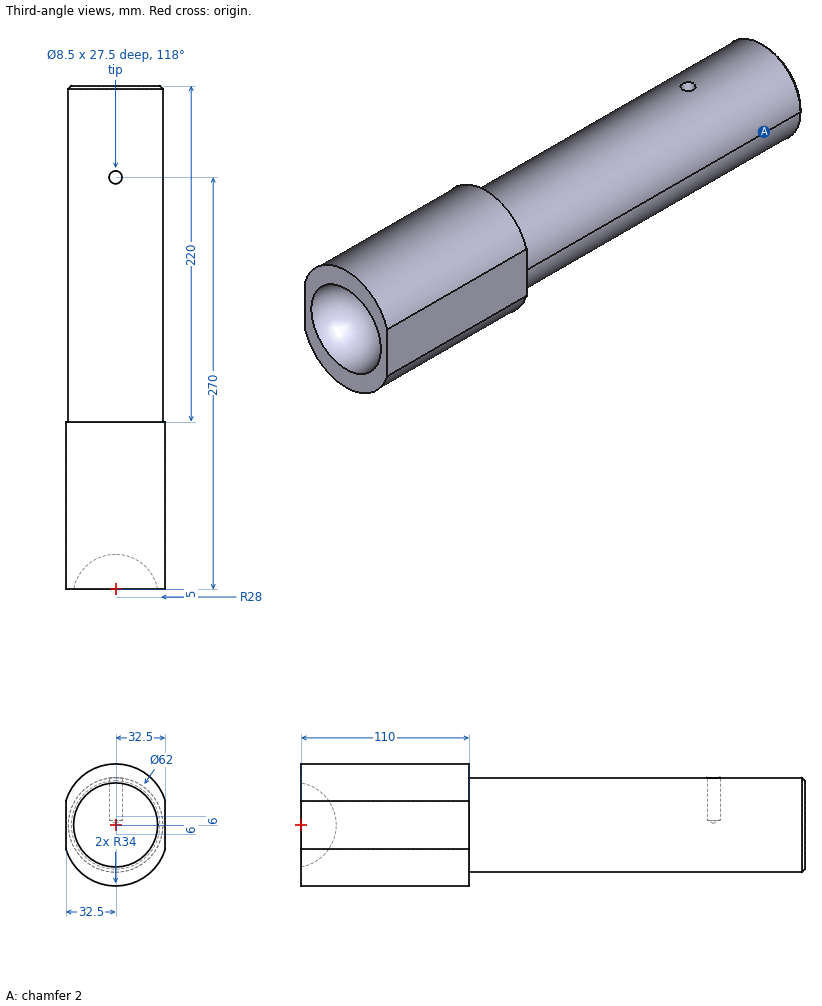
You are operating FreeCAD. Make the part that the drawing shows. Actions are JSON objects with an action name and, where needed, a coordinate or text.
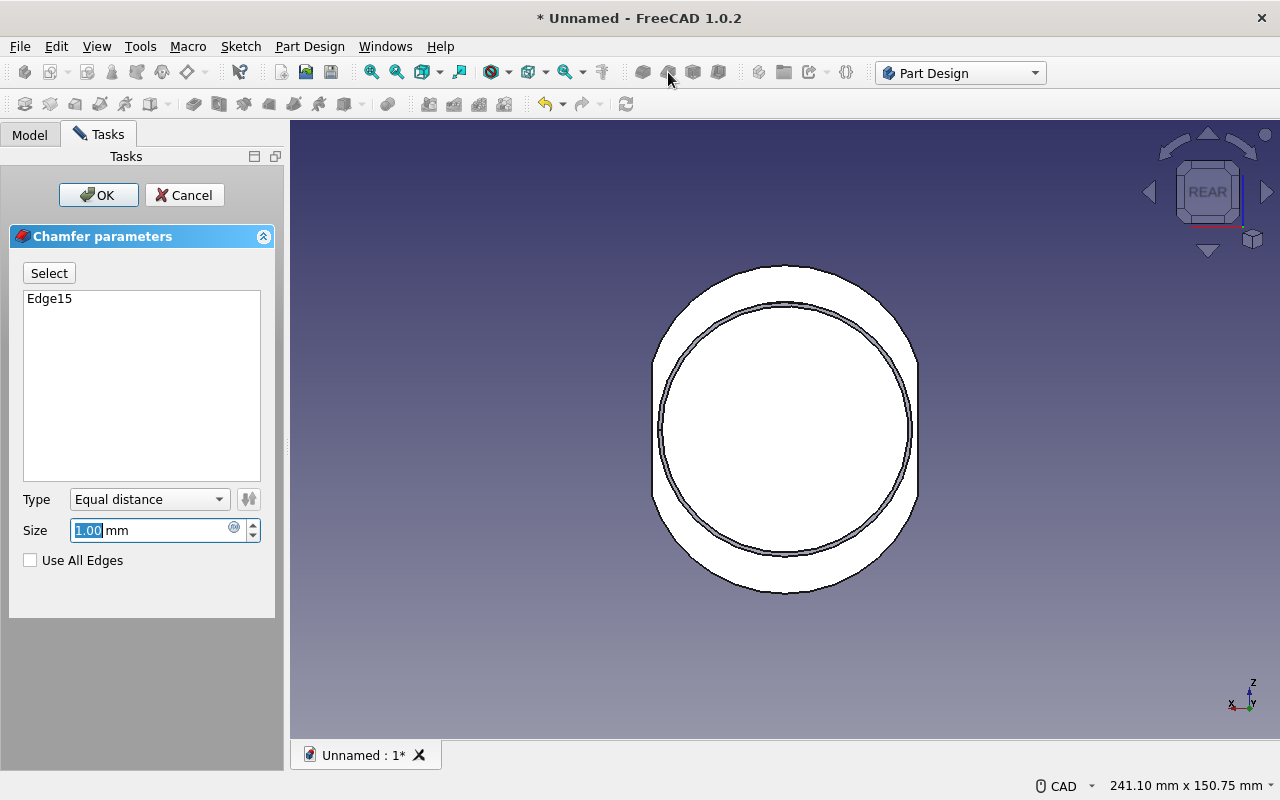
{"action": "type", "text": "2"}
{"action": "key", "text": "Tab"}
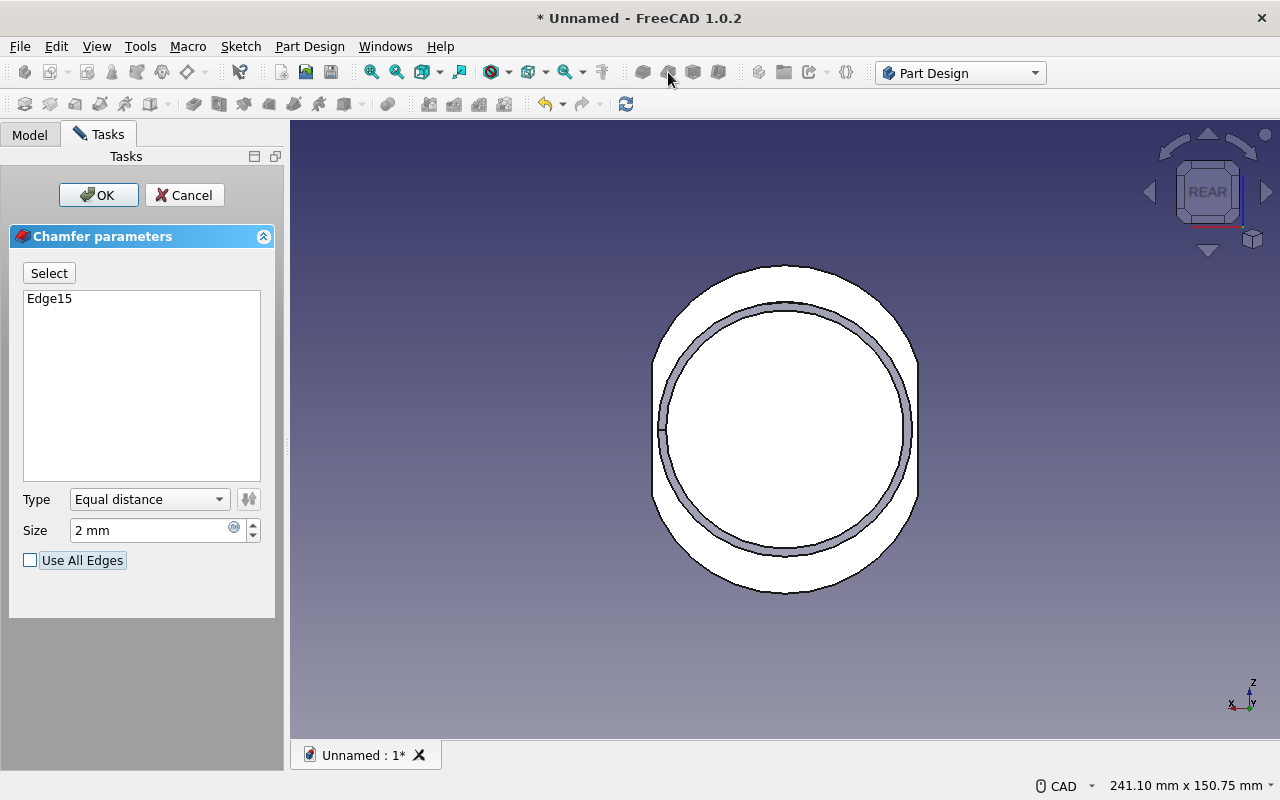
{"action": "left_click", "coordinate": [99, 195]}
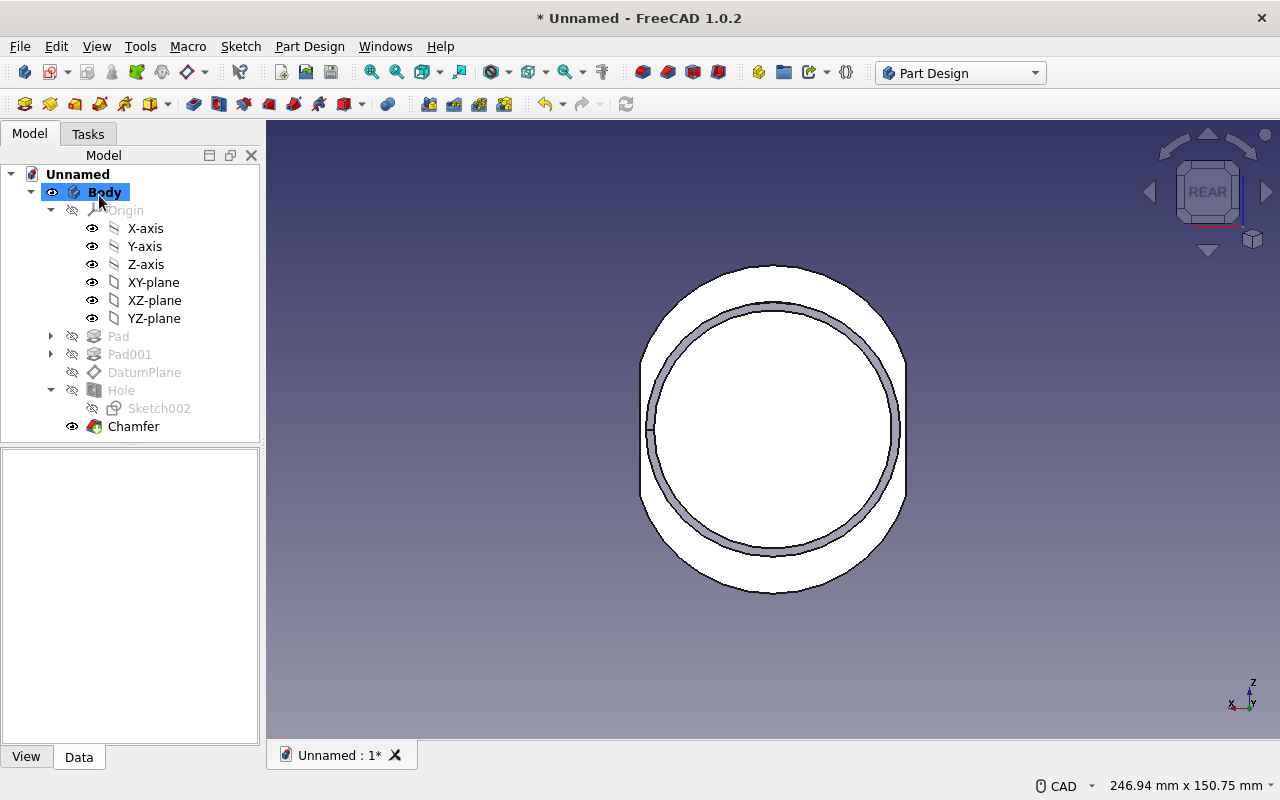
{"action": "left_click", "coordinate": [50, 72]}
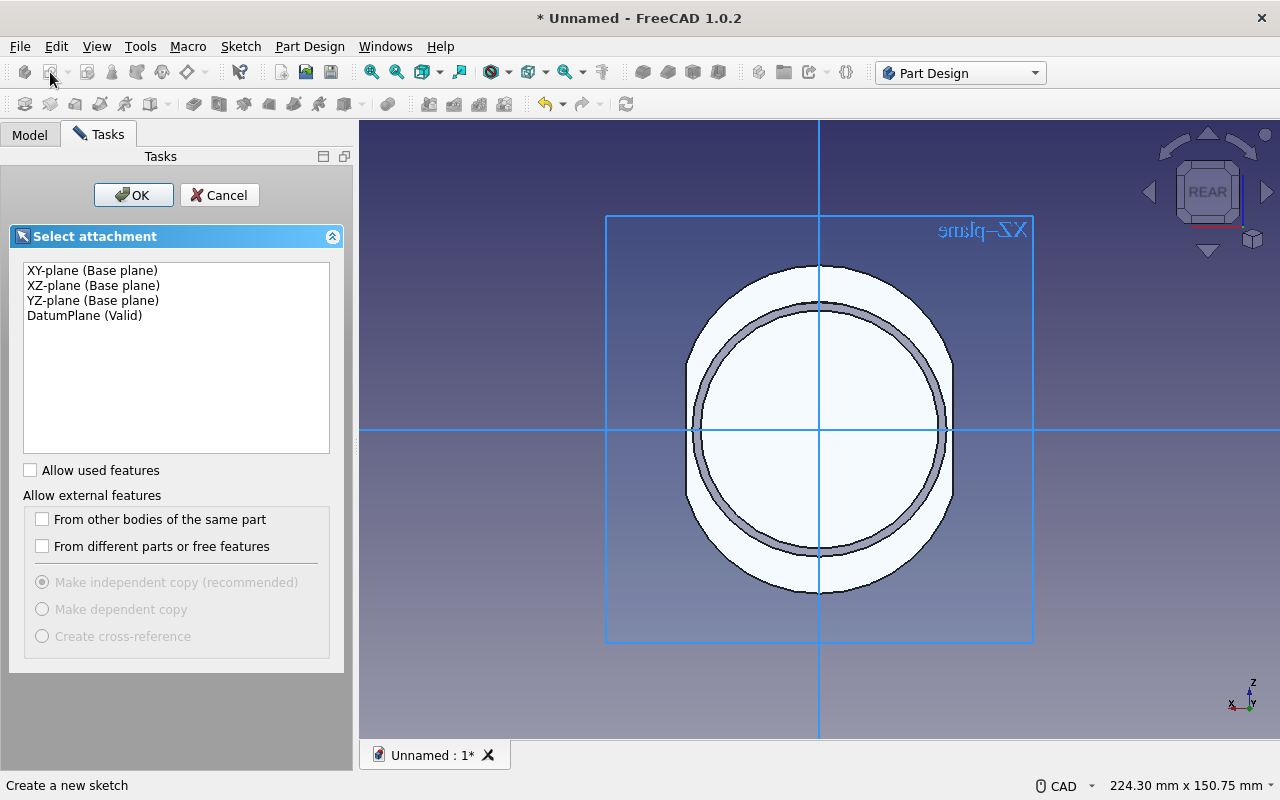
{"action": "left_click", "coordinate": [84, 270]}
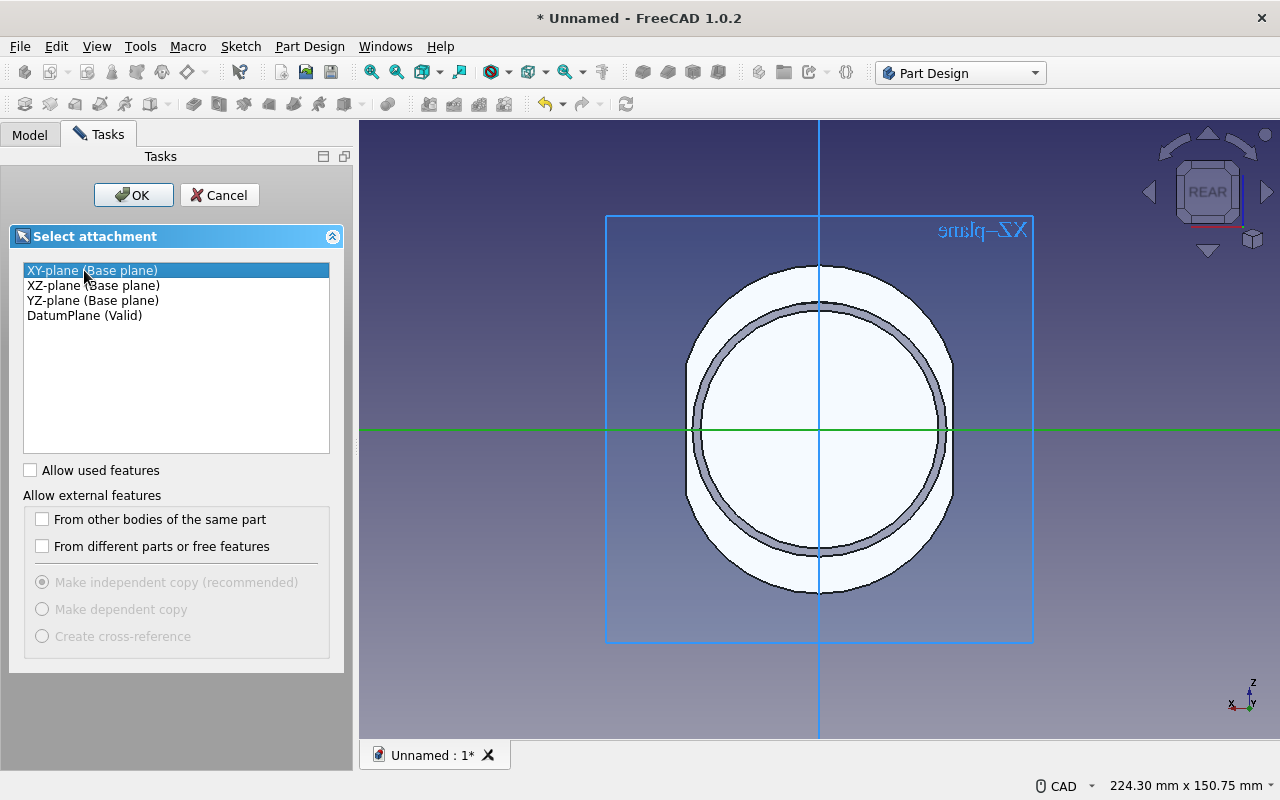
{"action": "left_click", "coordinate": [134, 195]}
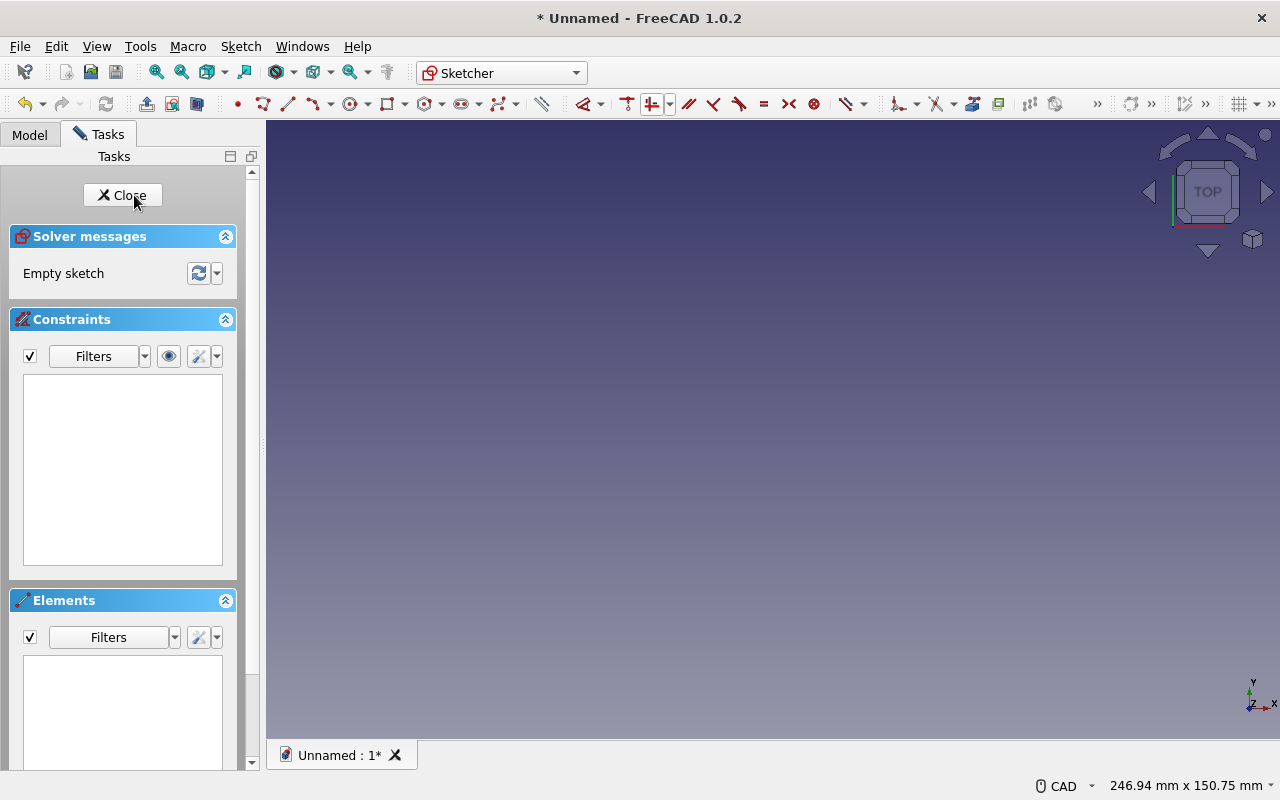
{"action": "left_click", "coordinate": [197, 104]}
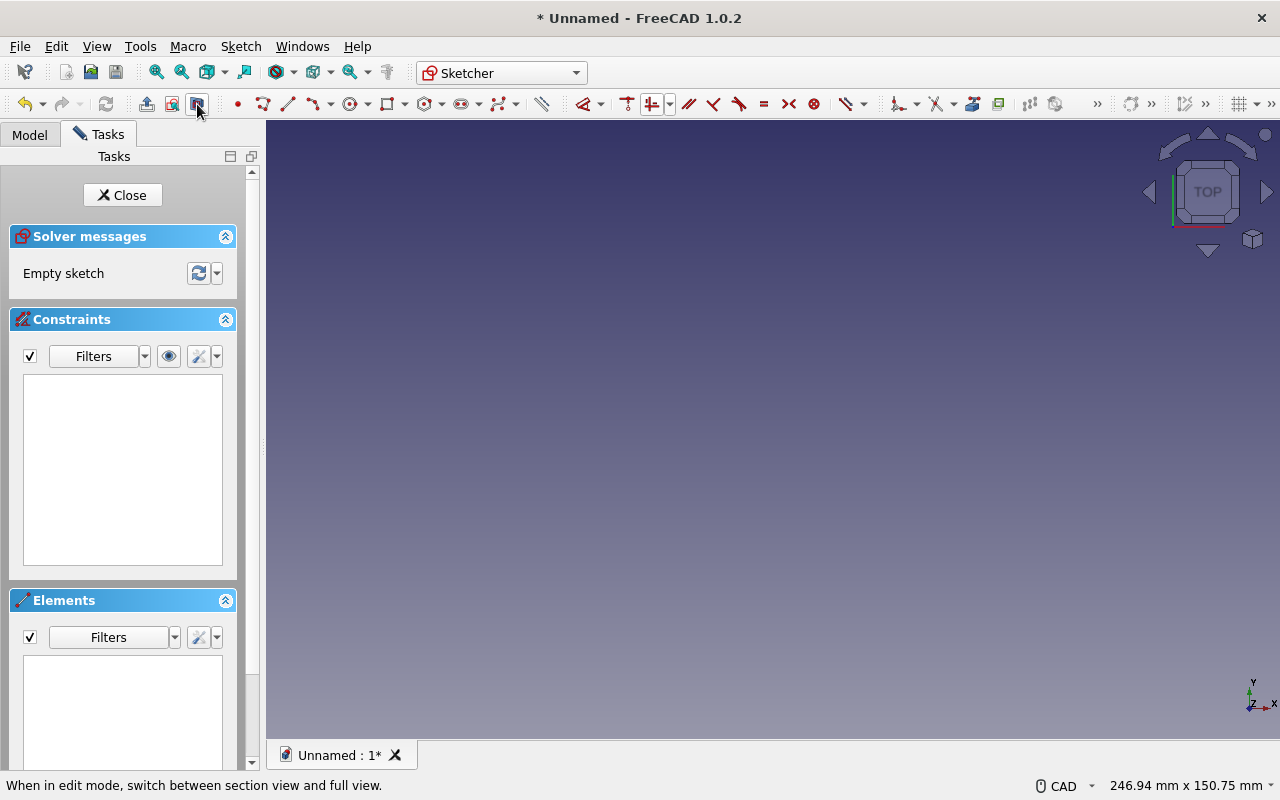
{"action": "scroll", "coordinate": [704, 430], "scroll_direction": "down", "scroll_amount": 5}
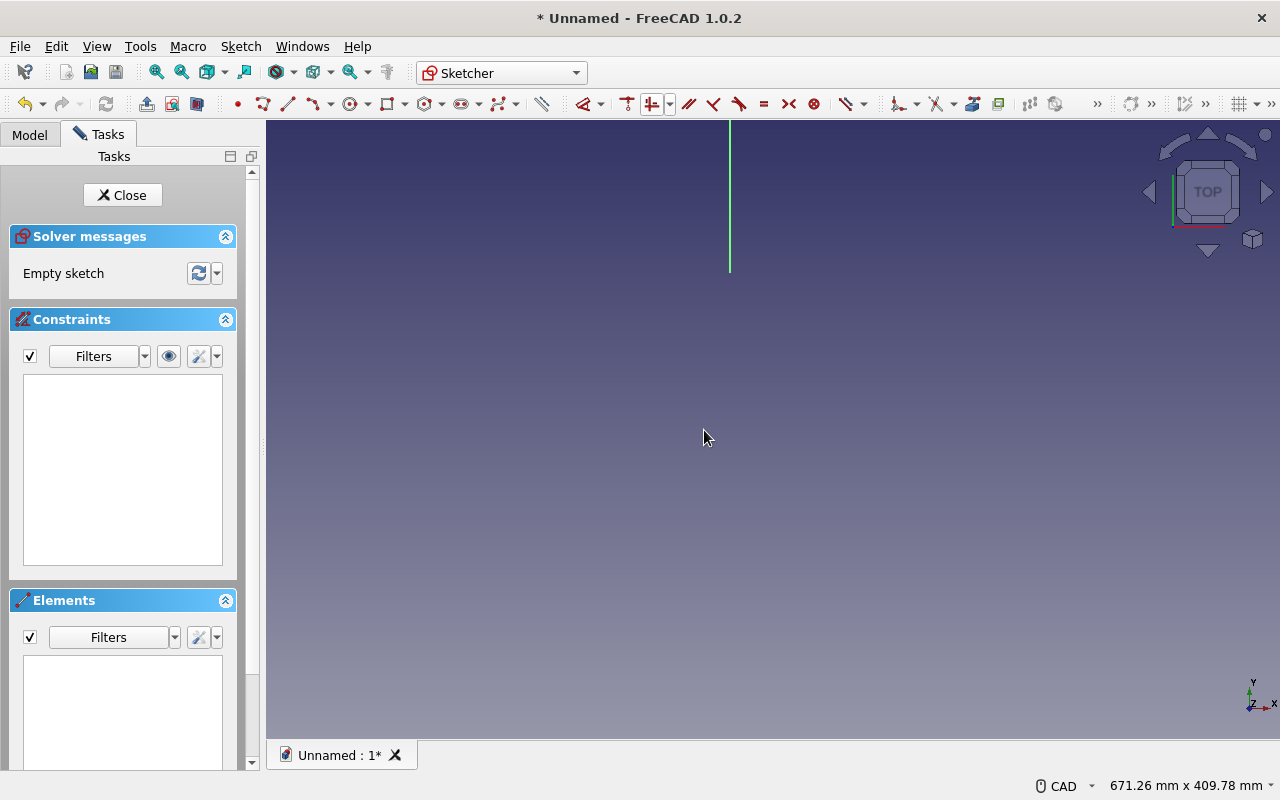
{"action": "scroll", "coordinate": [704, 430], "scroll_direction": "down", "scroll_amount": 5}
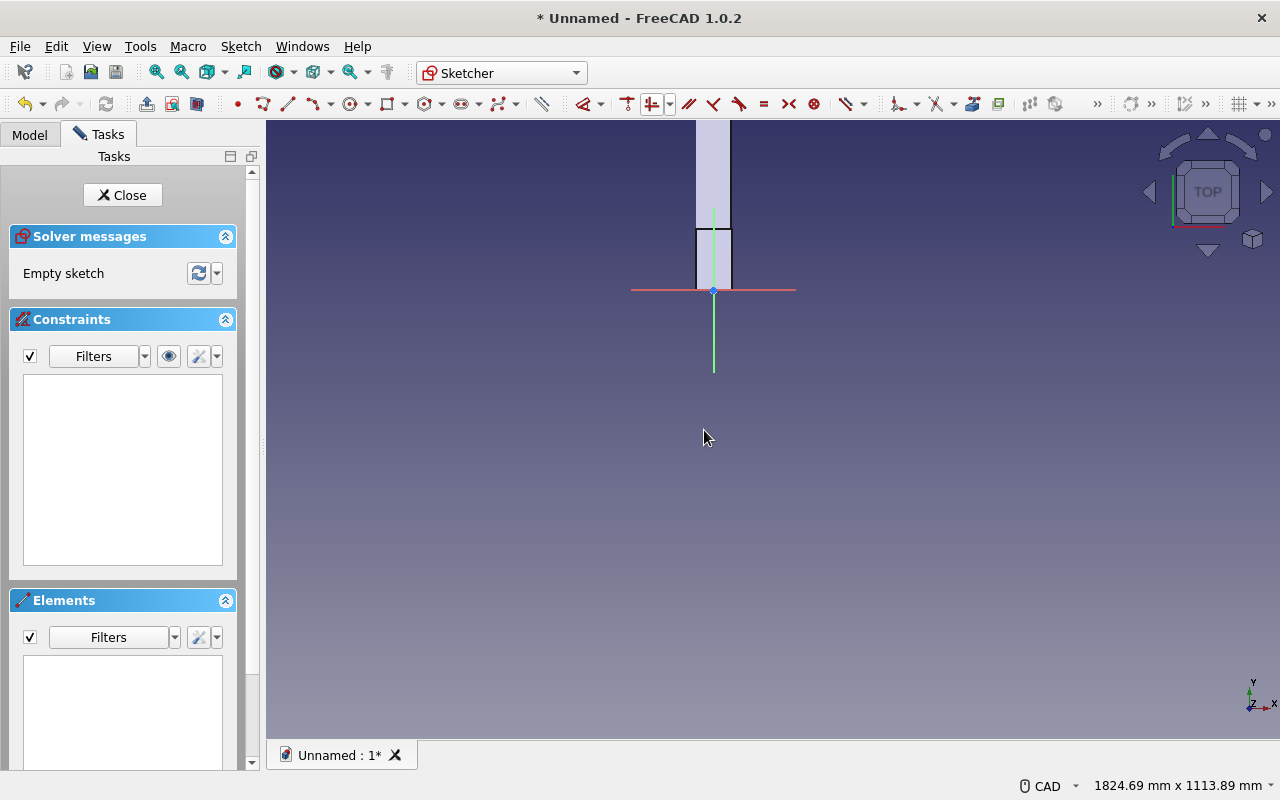
{"action": "scroll", "coordinate": [723, 282], "scroll_direction": "up", "scroll_amount": 13}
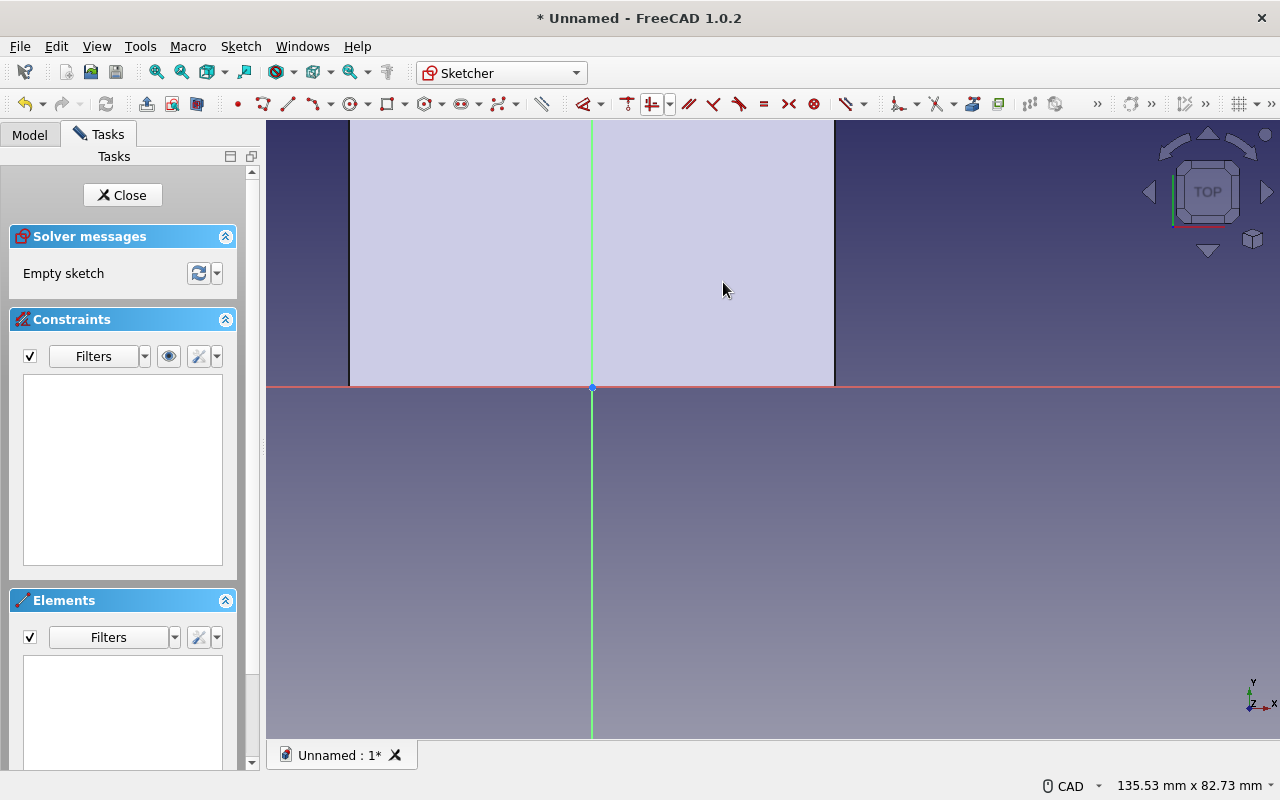
{"action": "left_click", "coordinate": [288, 104]}